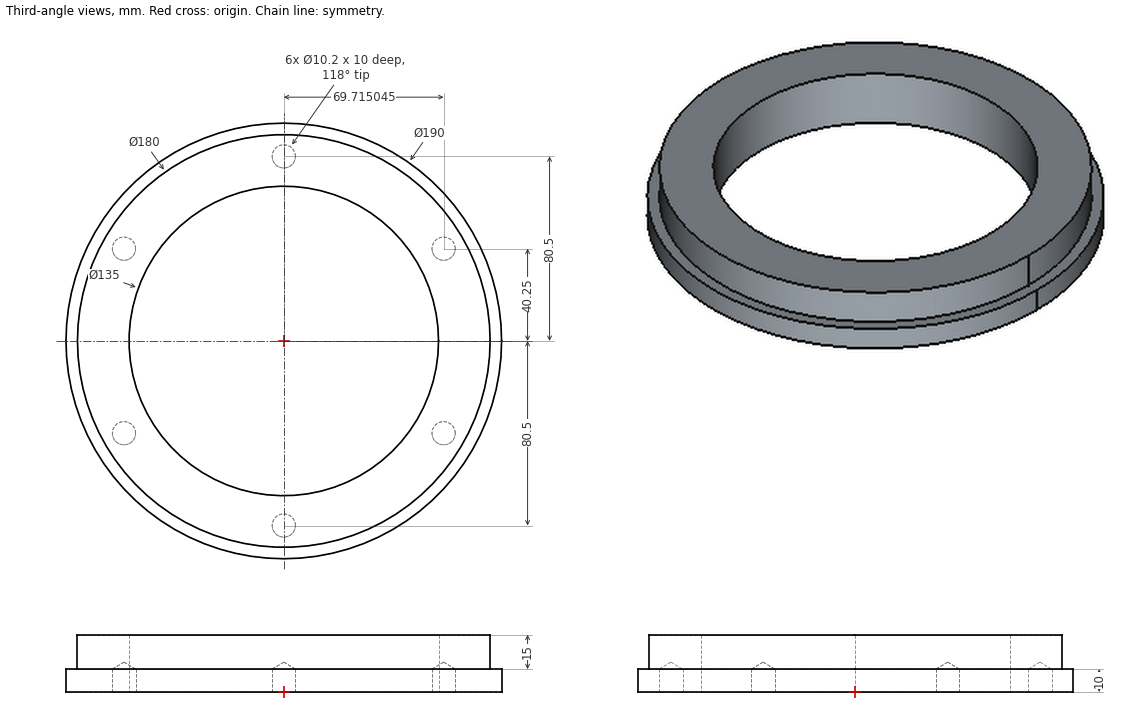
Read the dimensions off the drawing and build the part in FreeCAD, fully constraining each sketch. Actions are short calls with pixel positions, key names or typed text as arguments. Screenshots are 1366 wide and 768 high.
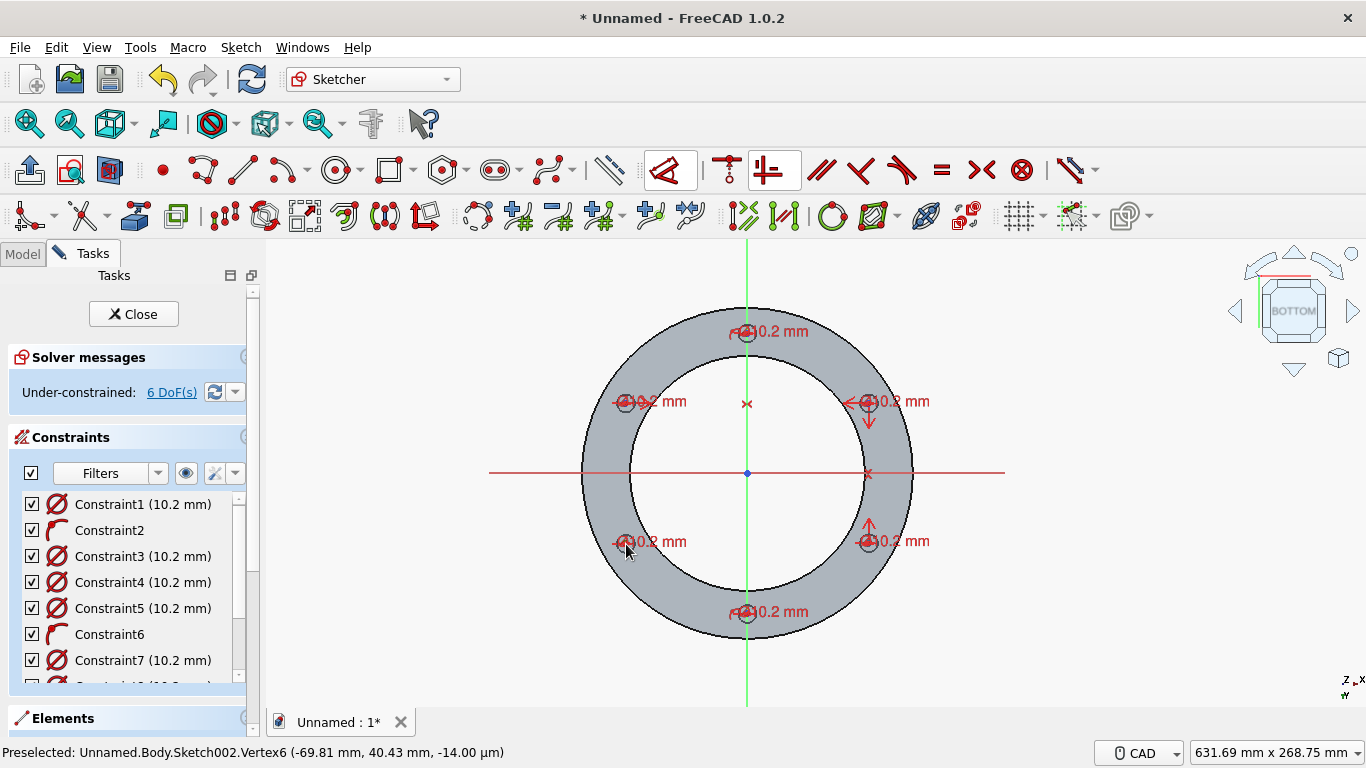
click(747, 561)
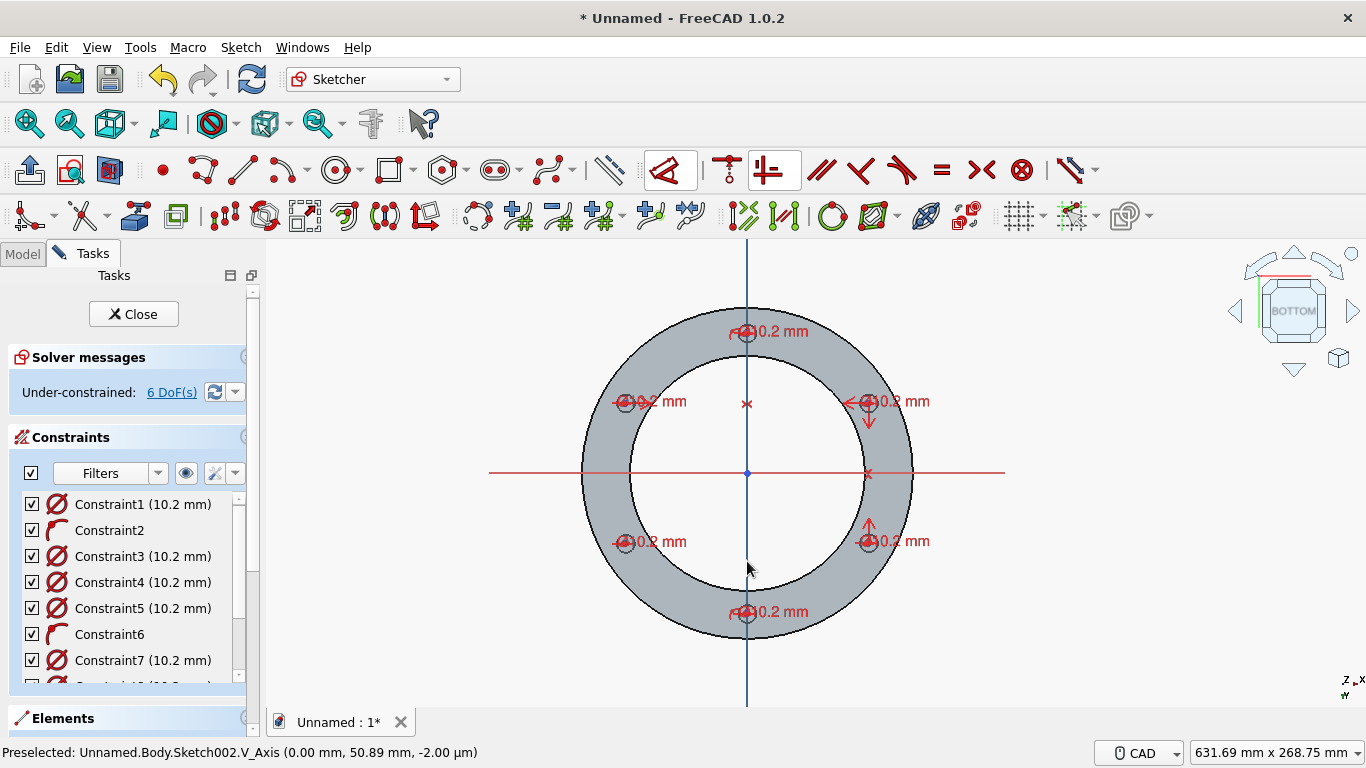
key(s)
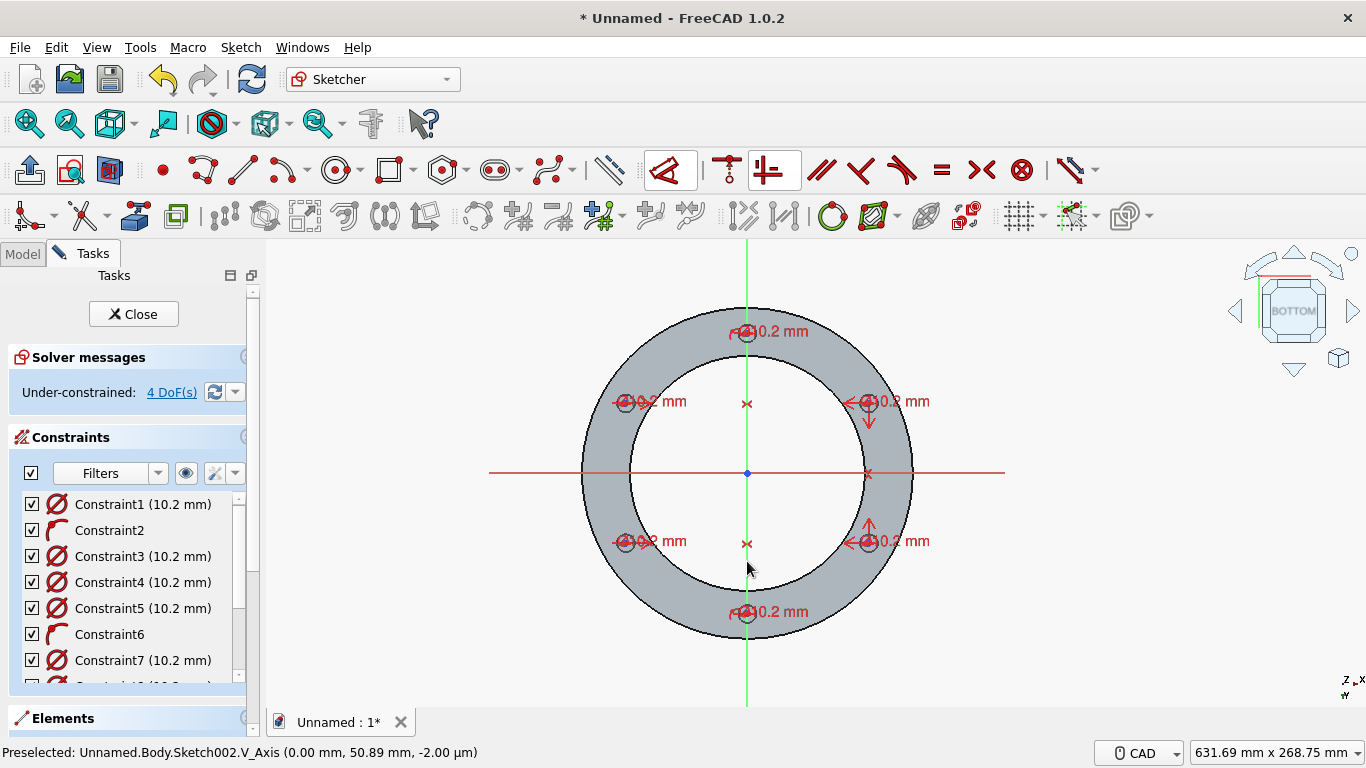
key(d)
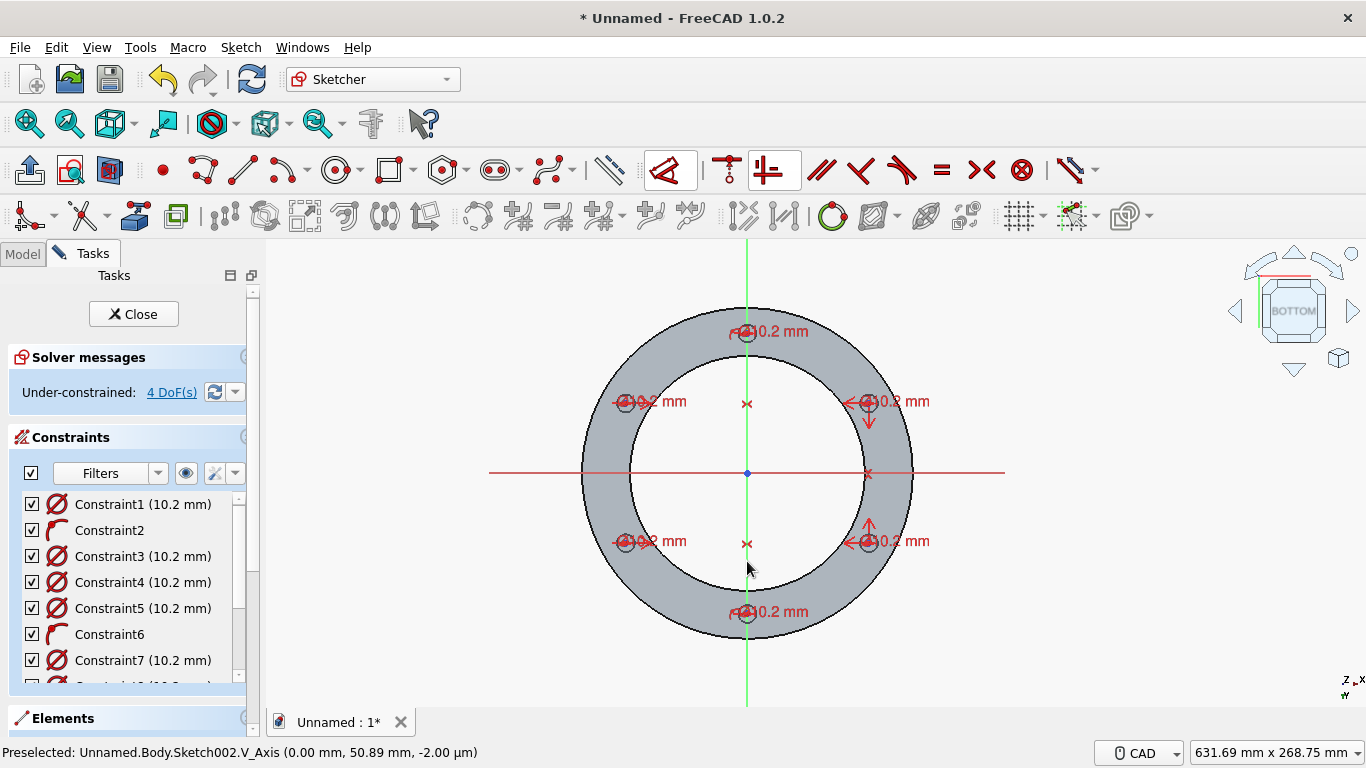
click(747, 614)
click(781, 544)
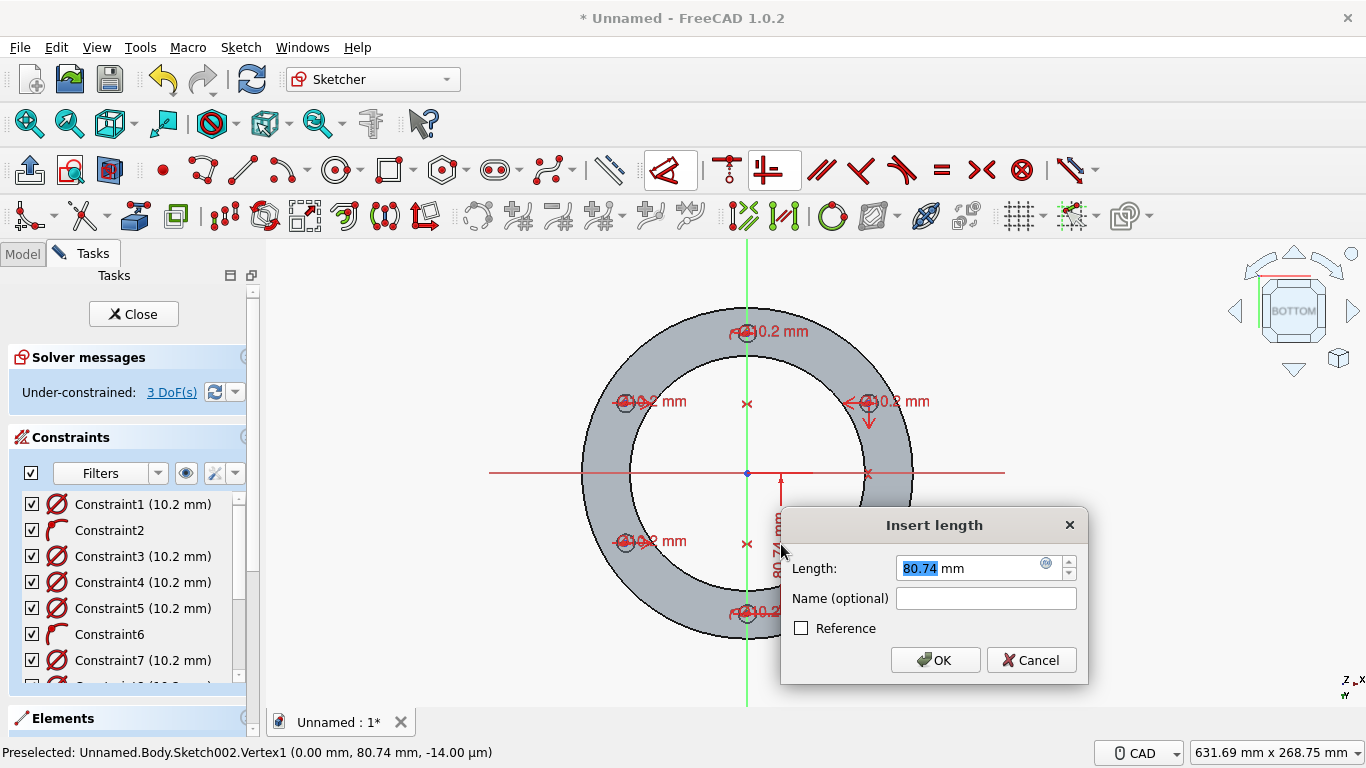
text(80.5)
key(Return)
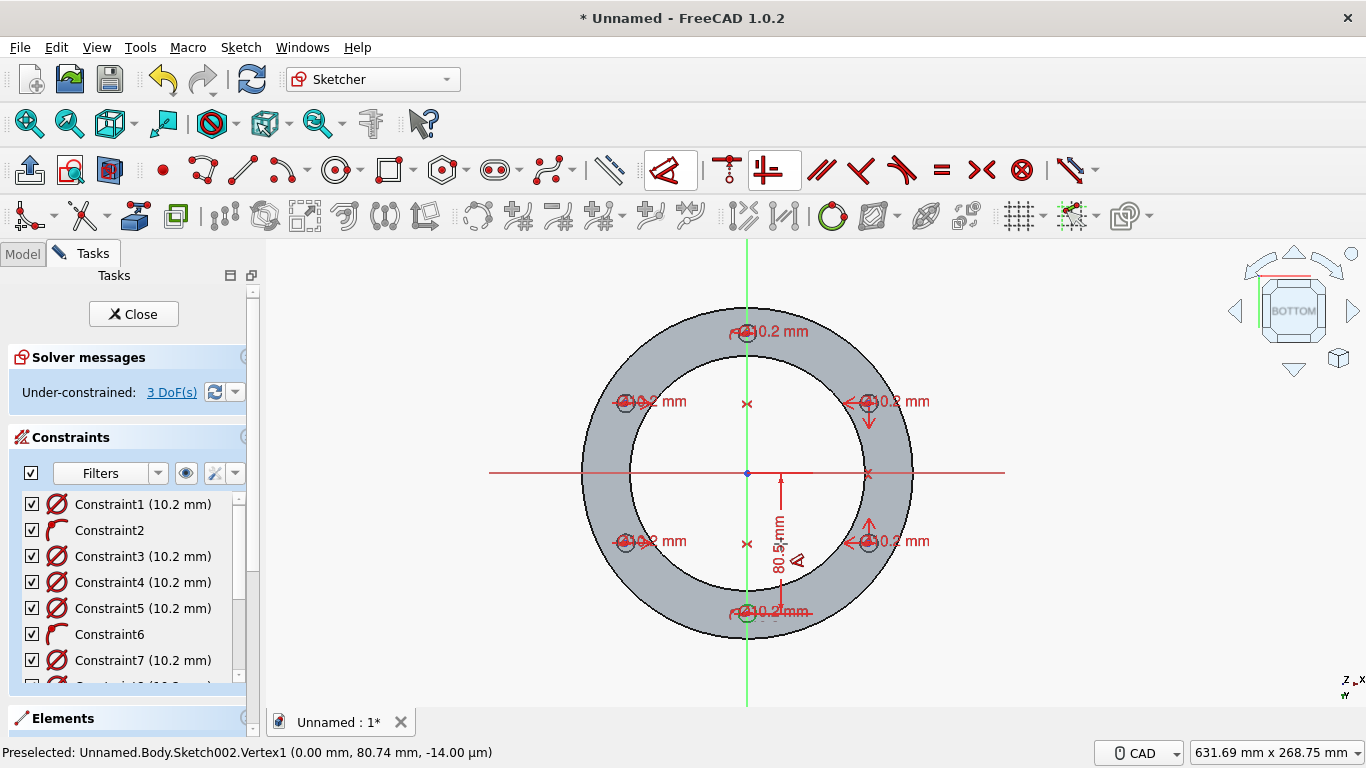
click(747, 333)
click(781, 403)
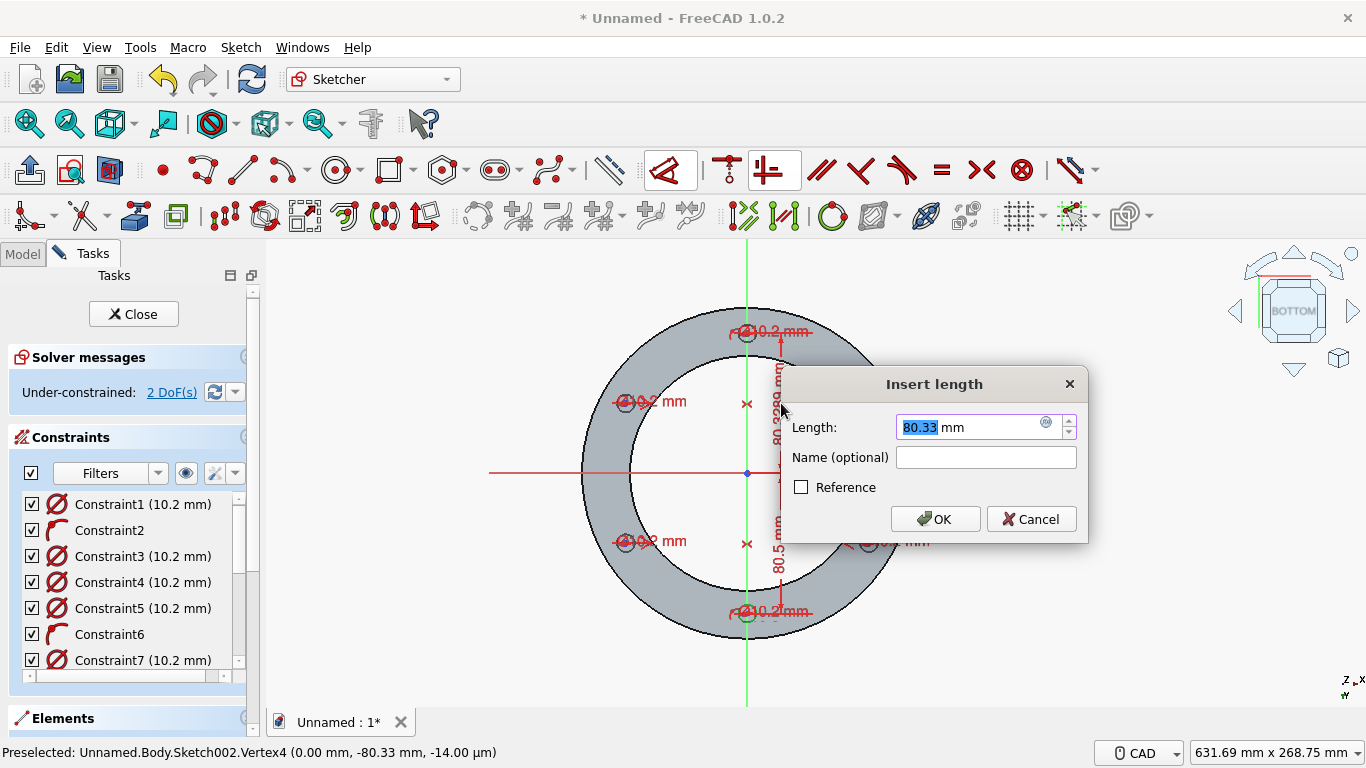
text(80.5)
key(Return)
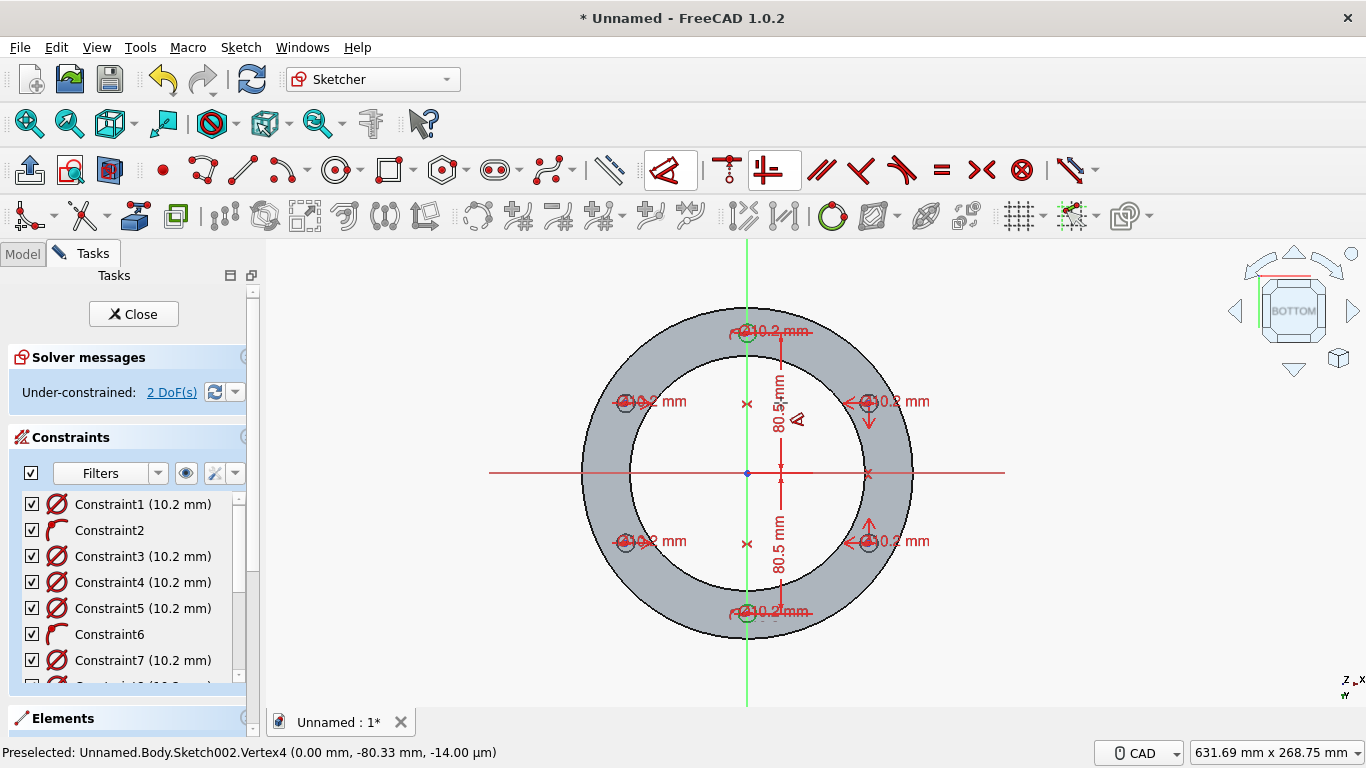
click(869, 543)
click(903, 508)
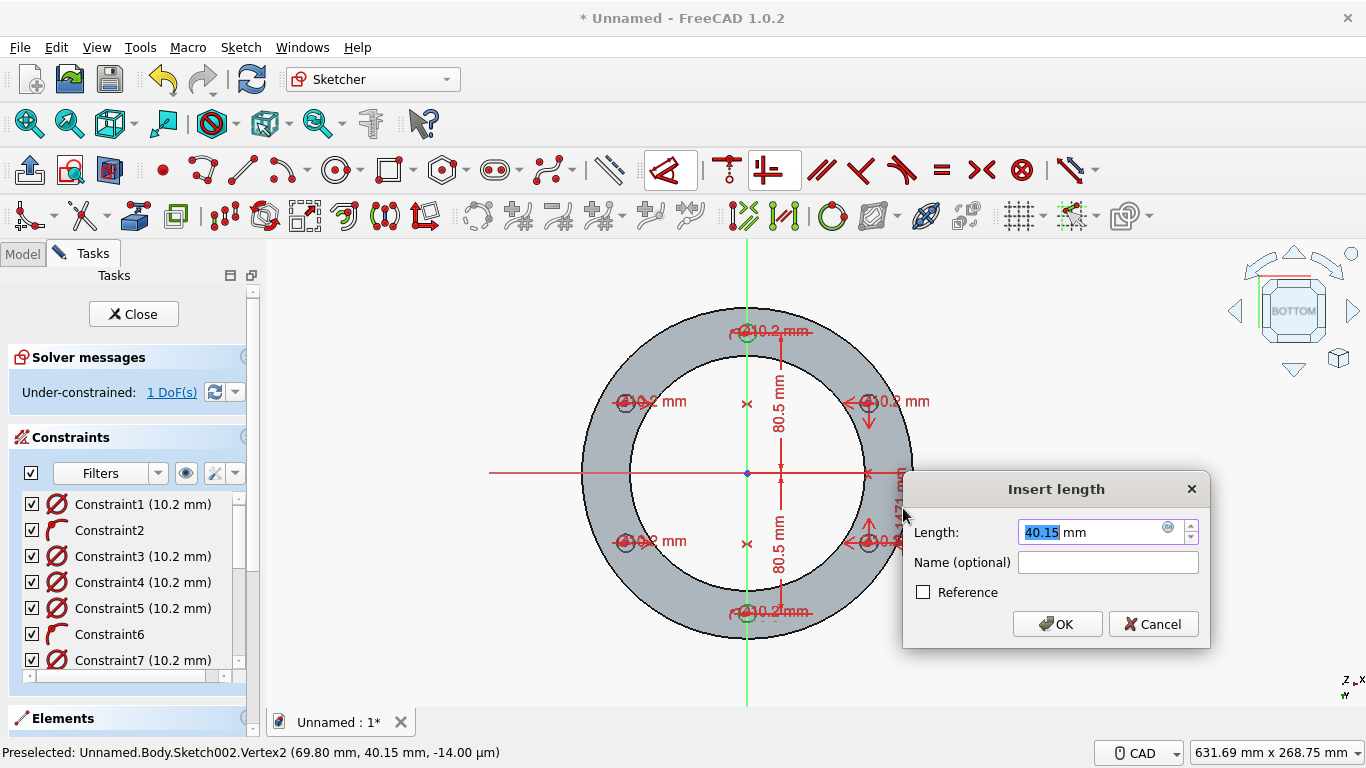
text(40.25)
key(Return)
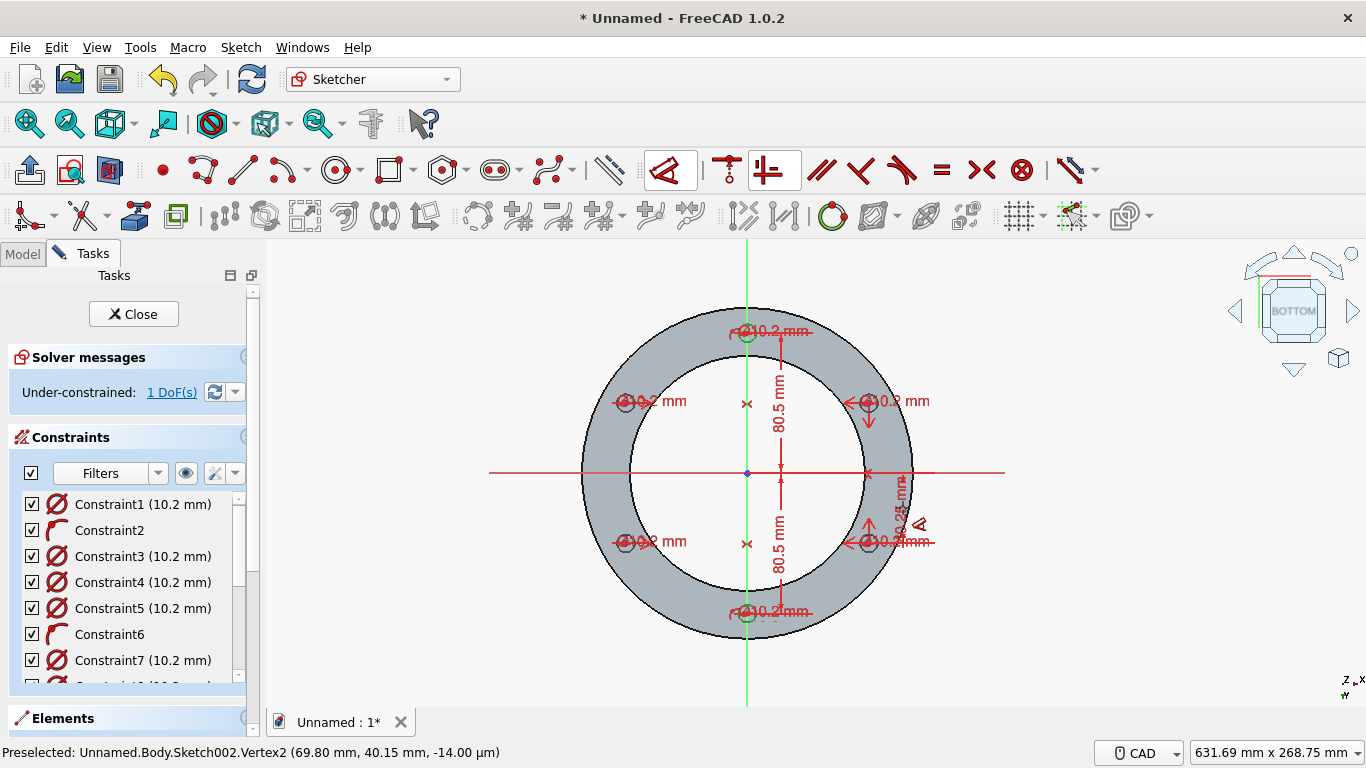
click(869, 543)
click(808, 577)